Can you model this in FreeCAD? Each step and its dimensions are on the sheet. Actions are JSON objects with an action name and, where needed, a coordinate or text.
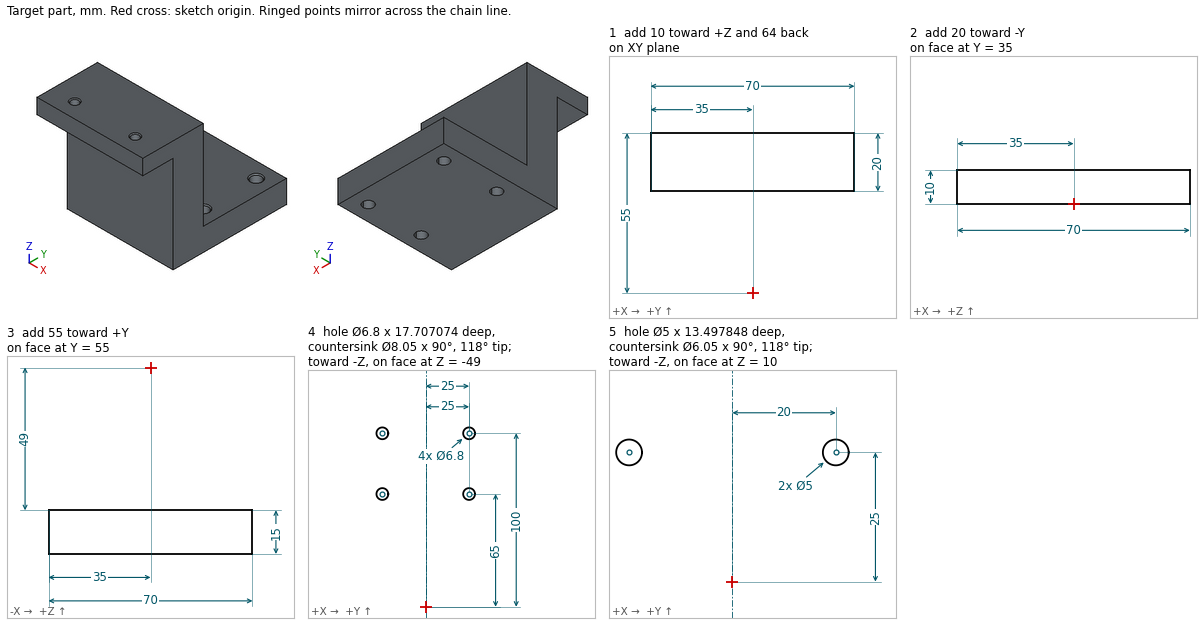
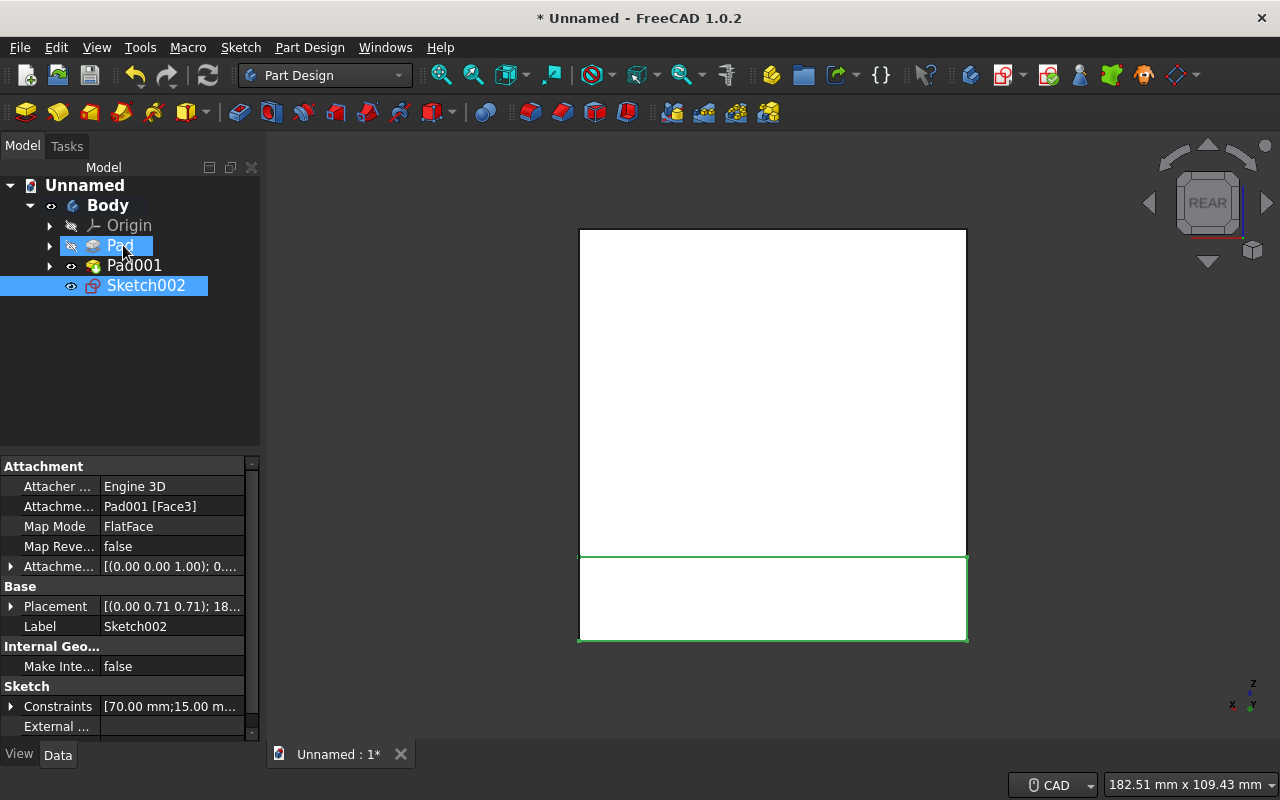
{"action": "left_click", "coordinate": [26, 112]}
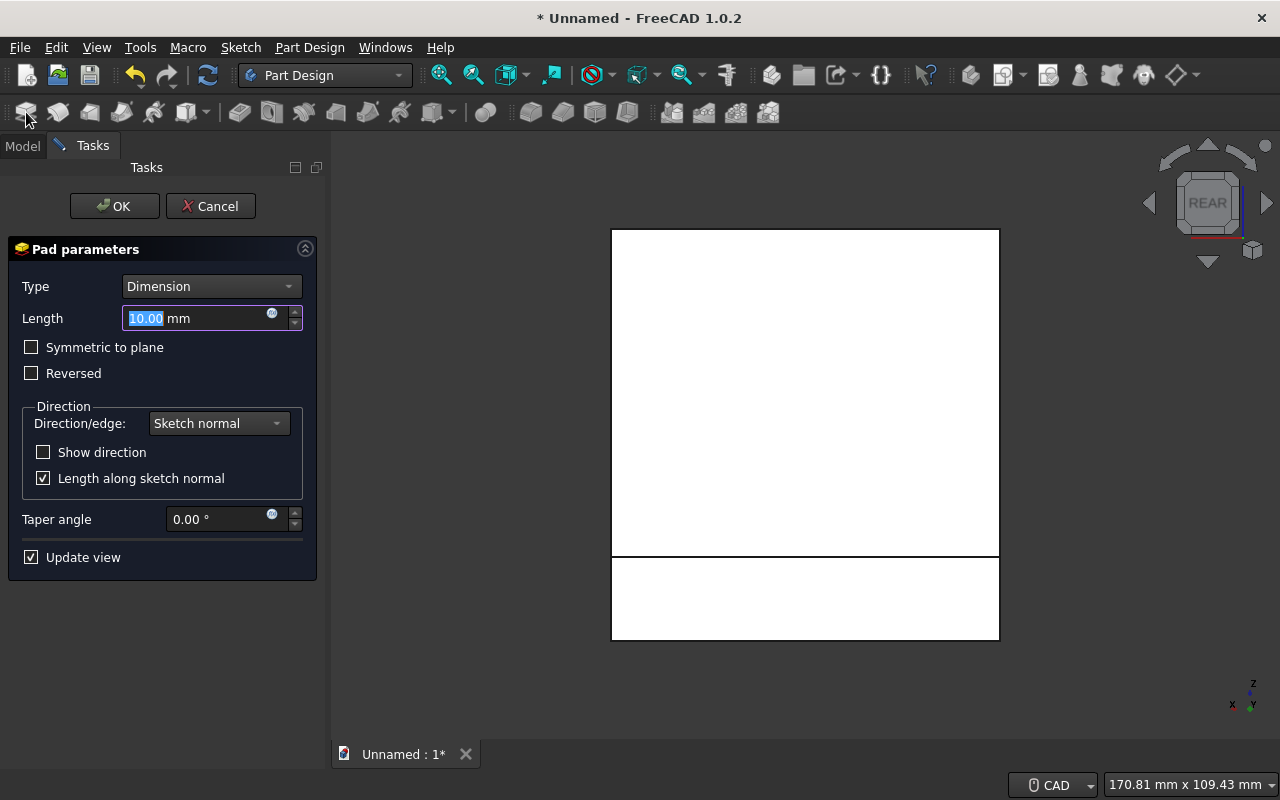
{"action": "type", "text": "55"}
{"action": "key", "text": "Tab"}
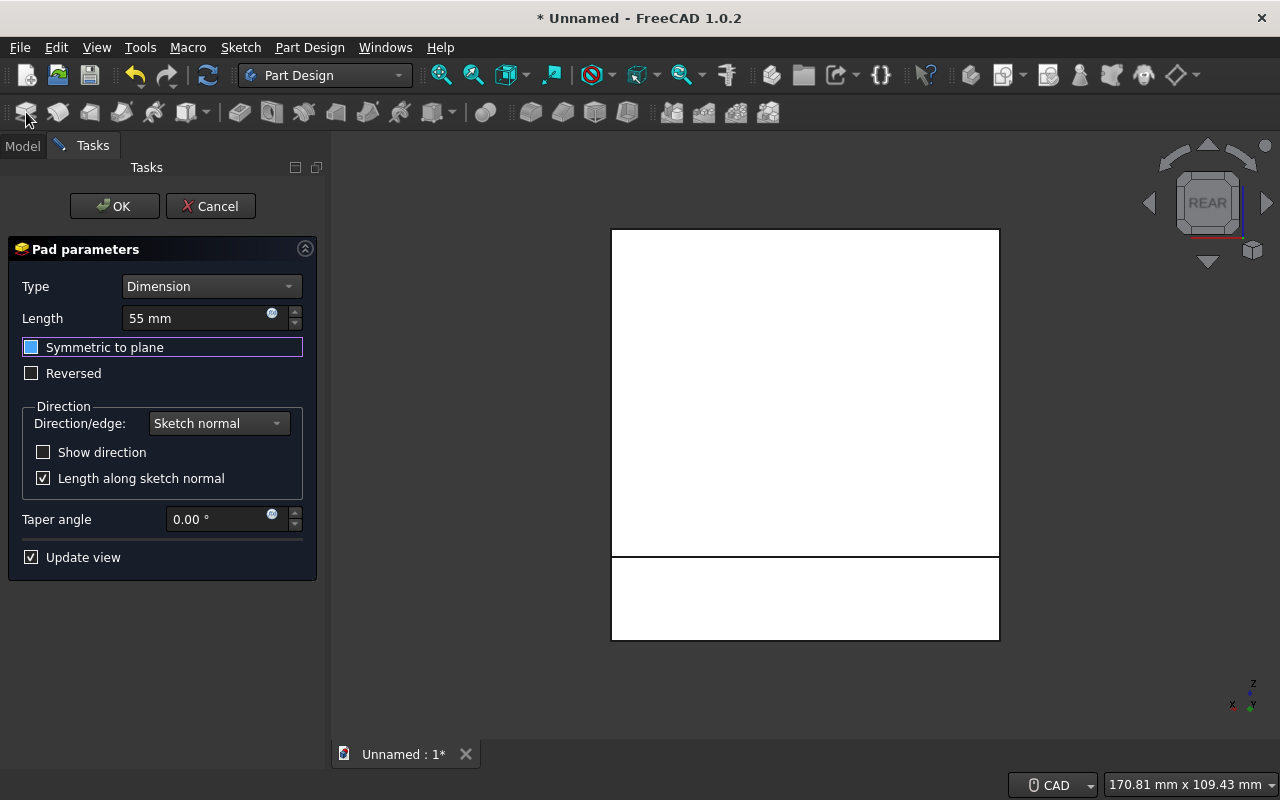
{"action": "left_click", "coordinate": [115, 206]}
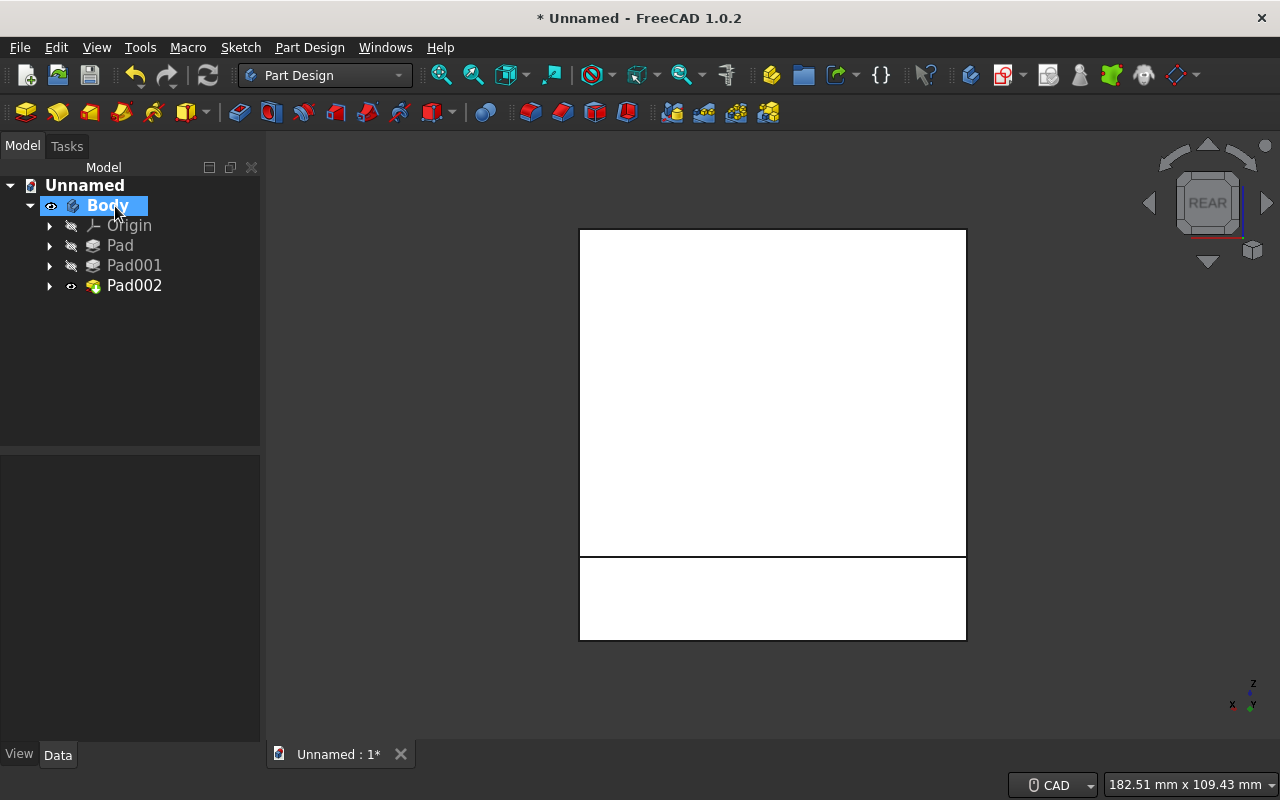
{"action": "key", "text": "0"}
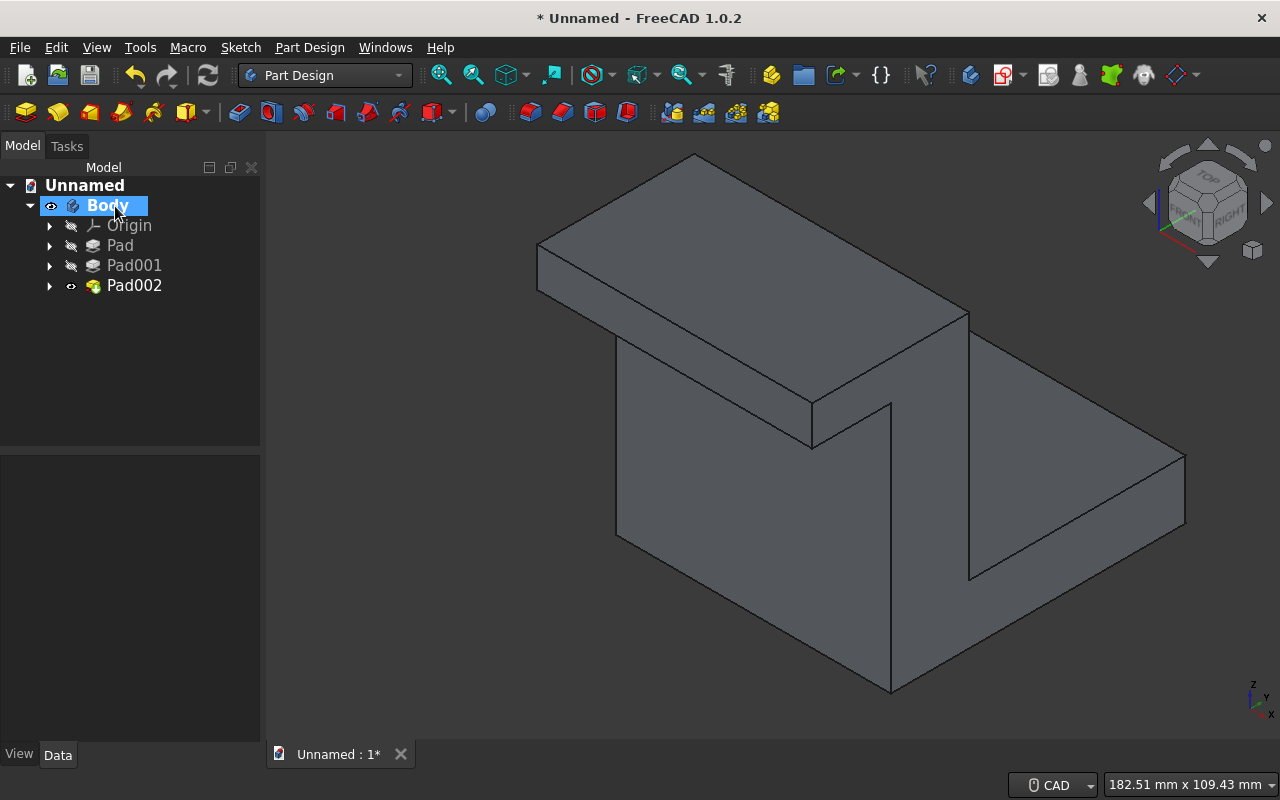
{"action": "key", "text": "v f"}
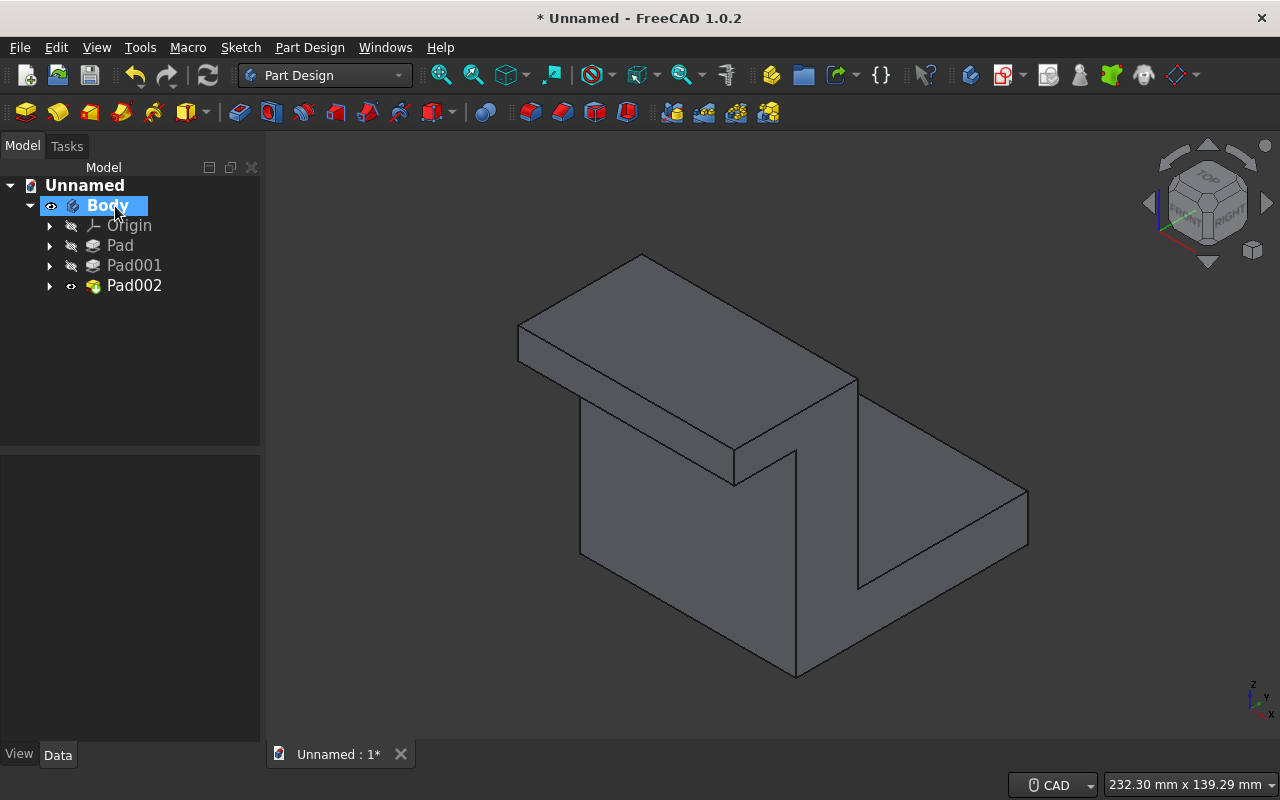
{"action": "left_click", "coordinate": [866, 495]}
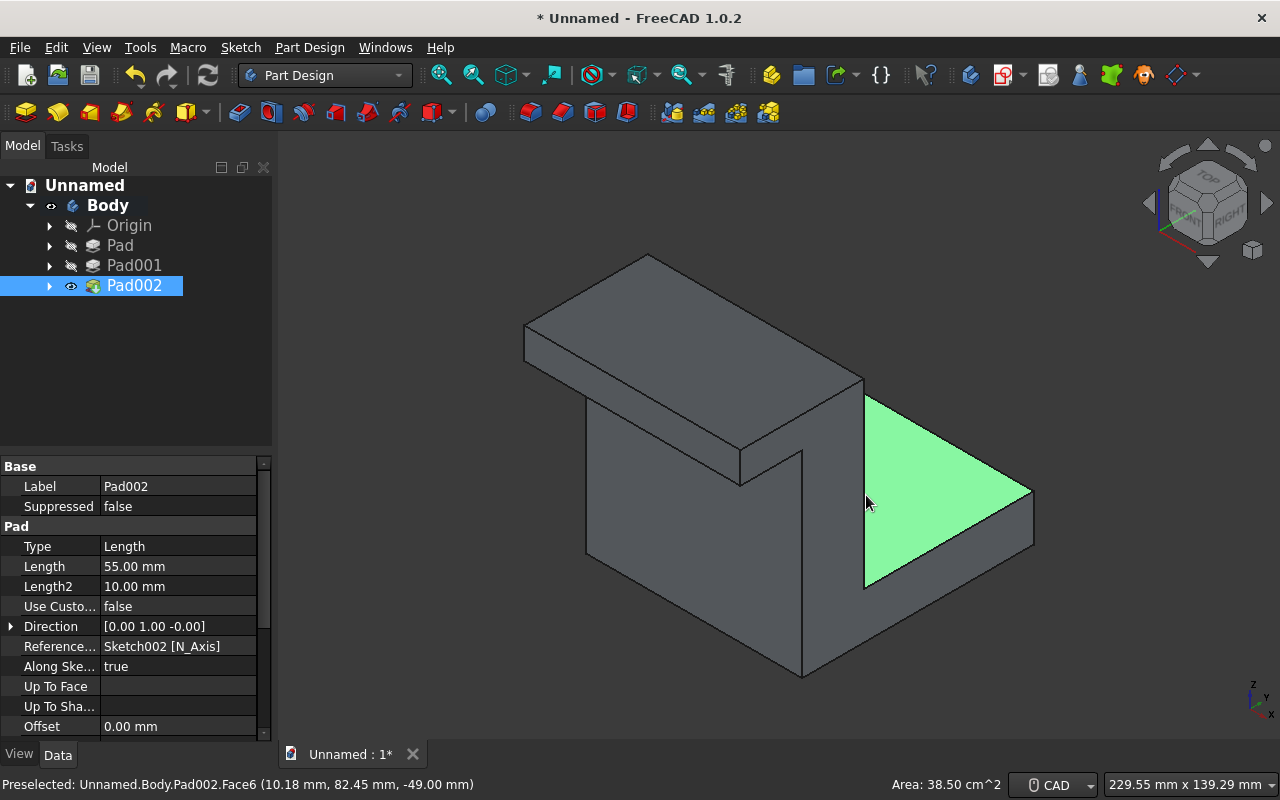
{"action": "left_click", "coordinate": [1004, 76]}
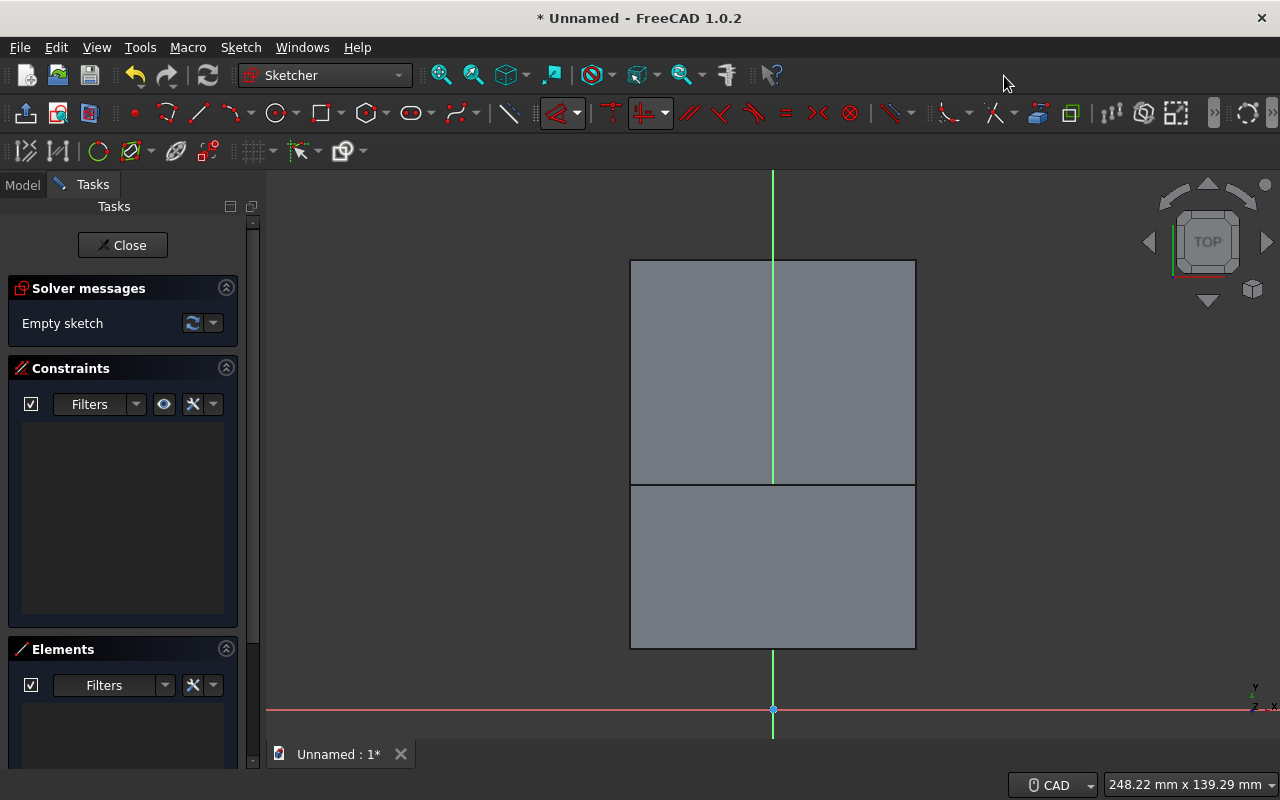
{"action": "scroll", "coordinate": [395, 255], "scroll_direction": "down", "scroll_amount": 1}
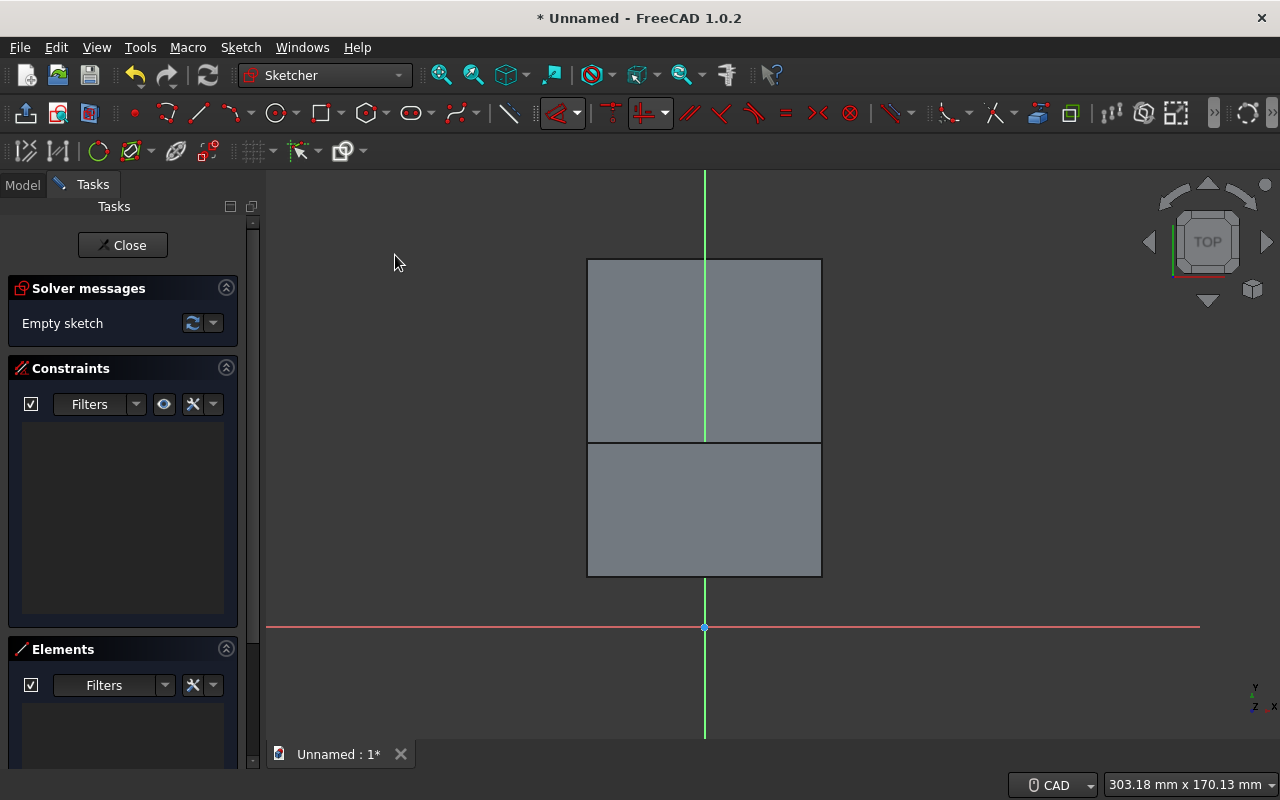
{"action": "left_click", "coordinate": [276, 114]}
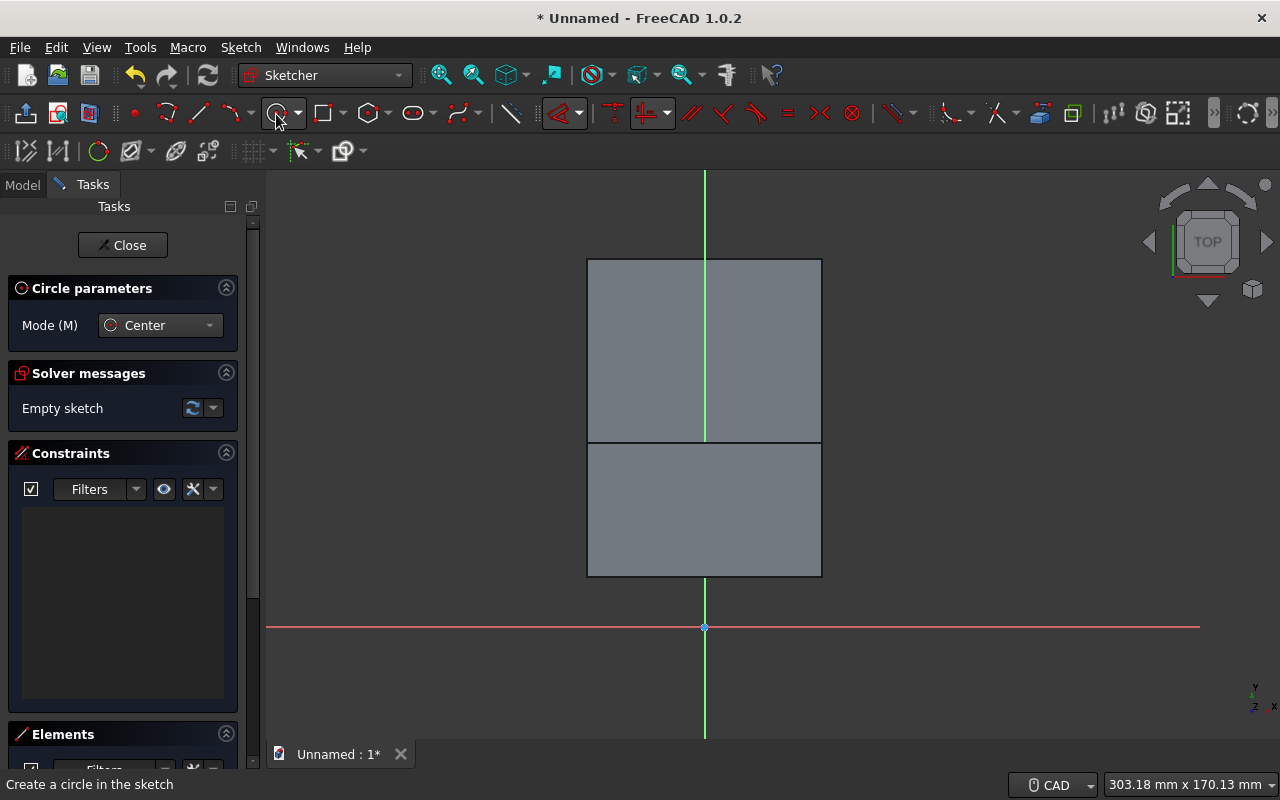
{"action": "scroll", "coordinate": [788, 293], "scroll_direction": "up", "scroll_amount": 4}